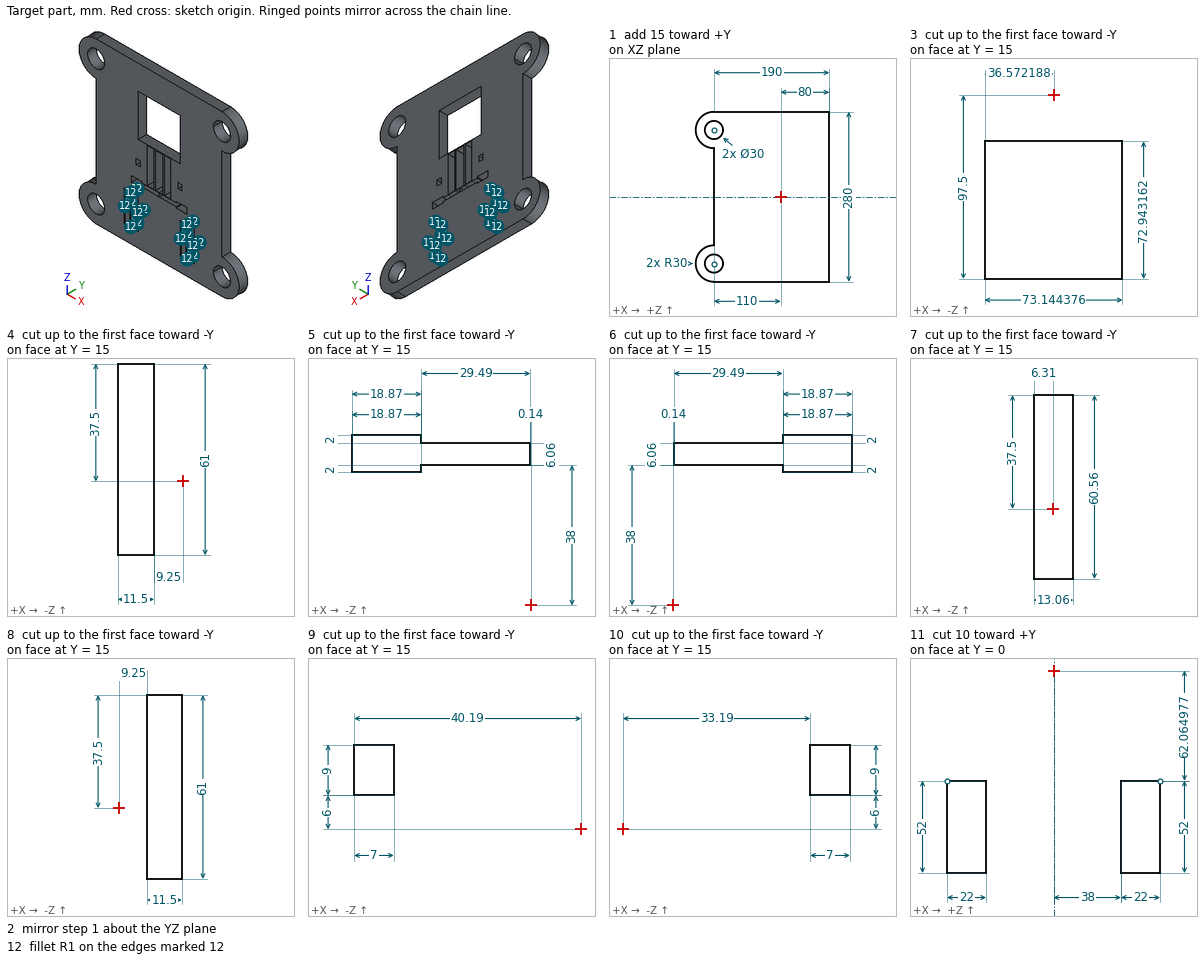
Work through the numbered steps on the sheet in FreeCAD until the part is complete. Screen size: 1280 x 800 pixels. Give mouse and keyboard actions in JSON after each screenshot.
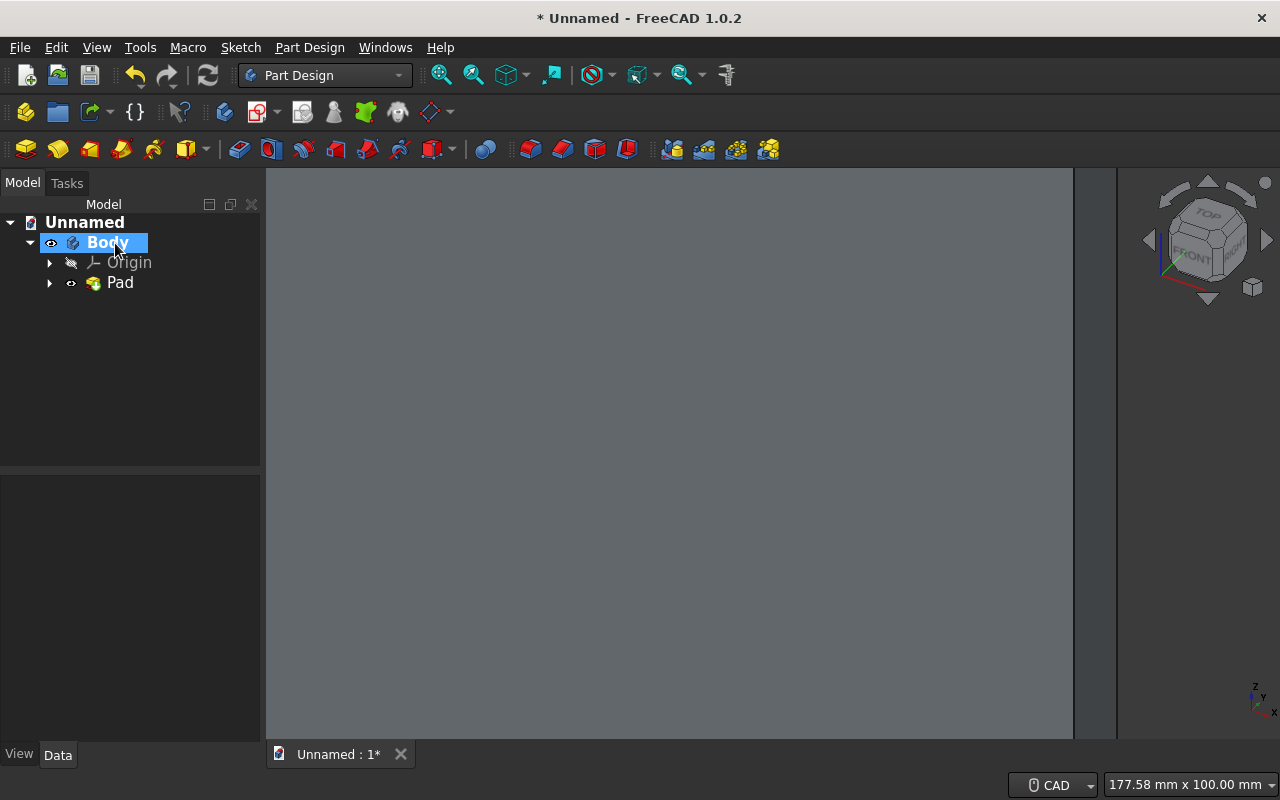
{"action": "left_click", "coordinate": [442, 76]}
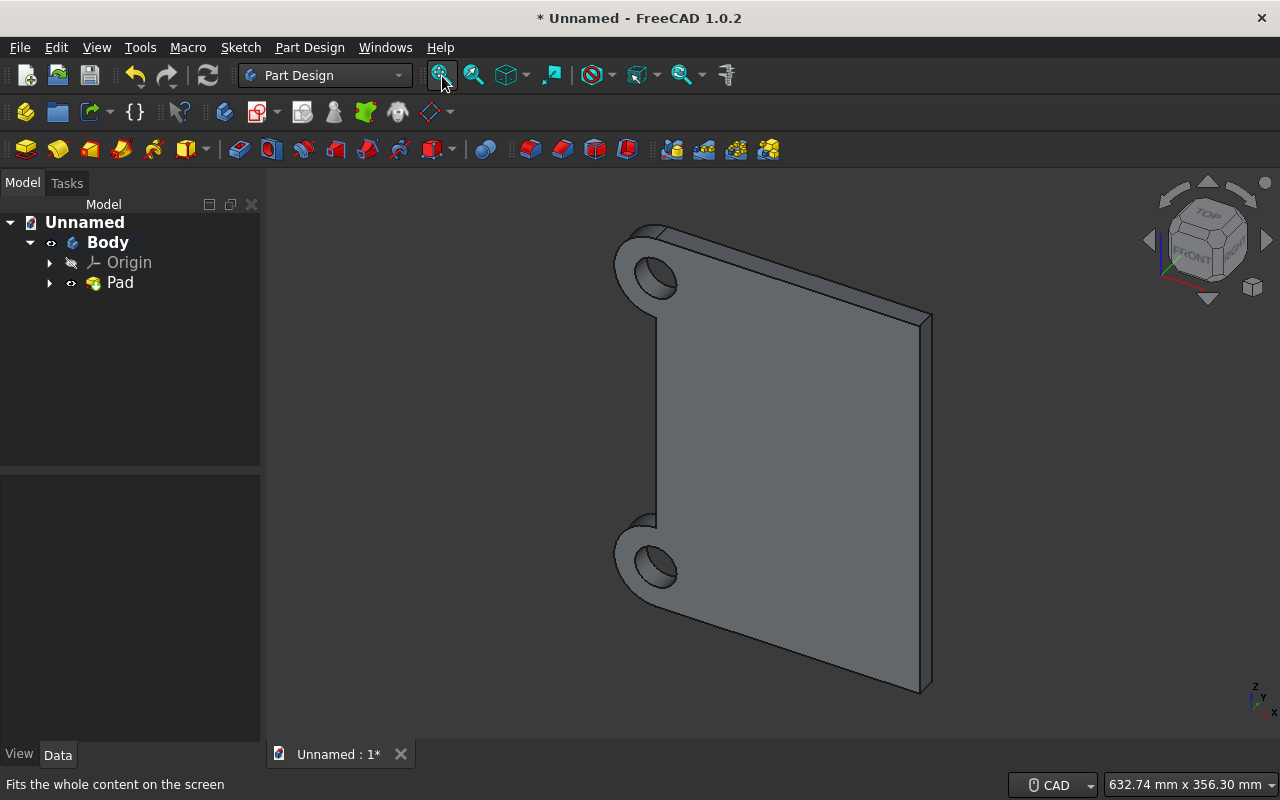
{"action": "left_click", "coordinate": [116, 283]}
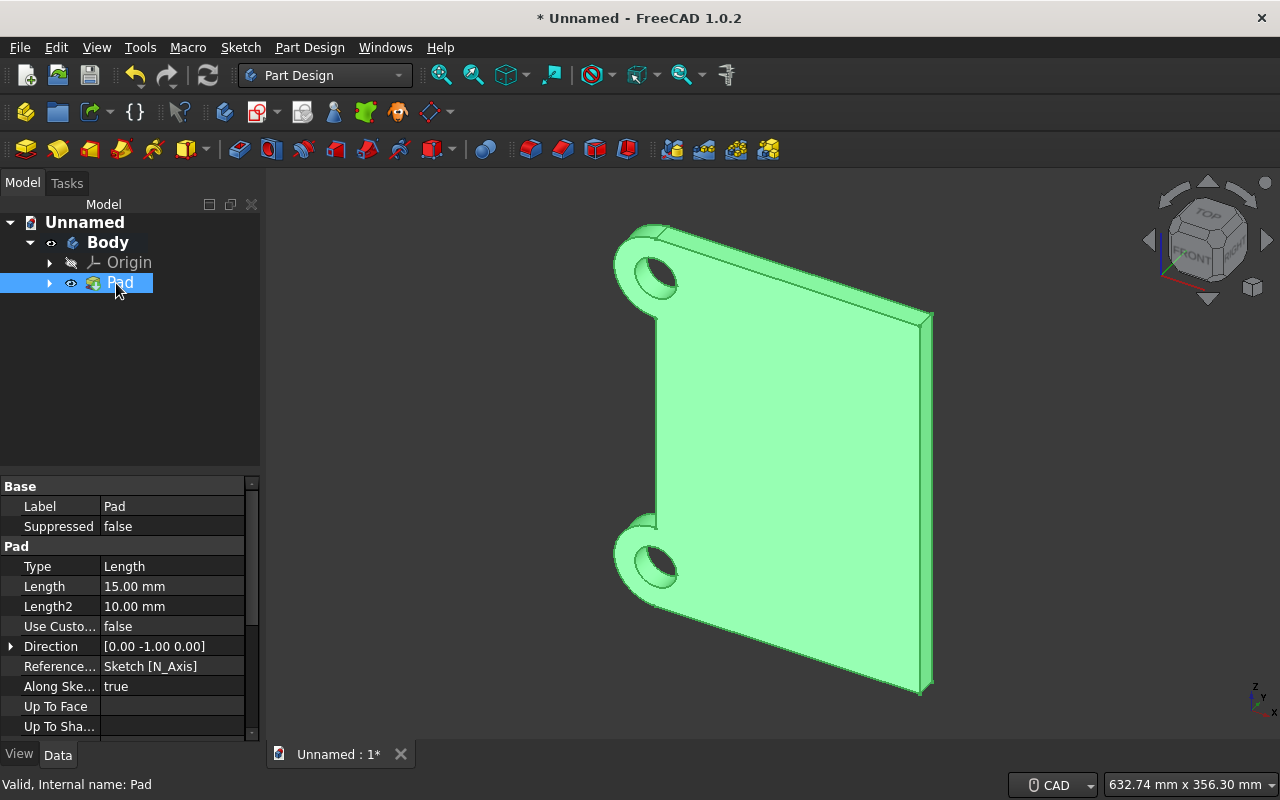
{"action": "left_click", "coordinate": [672, 150]}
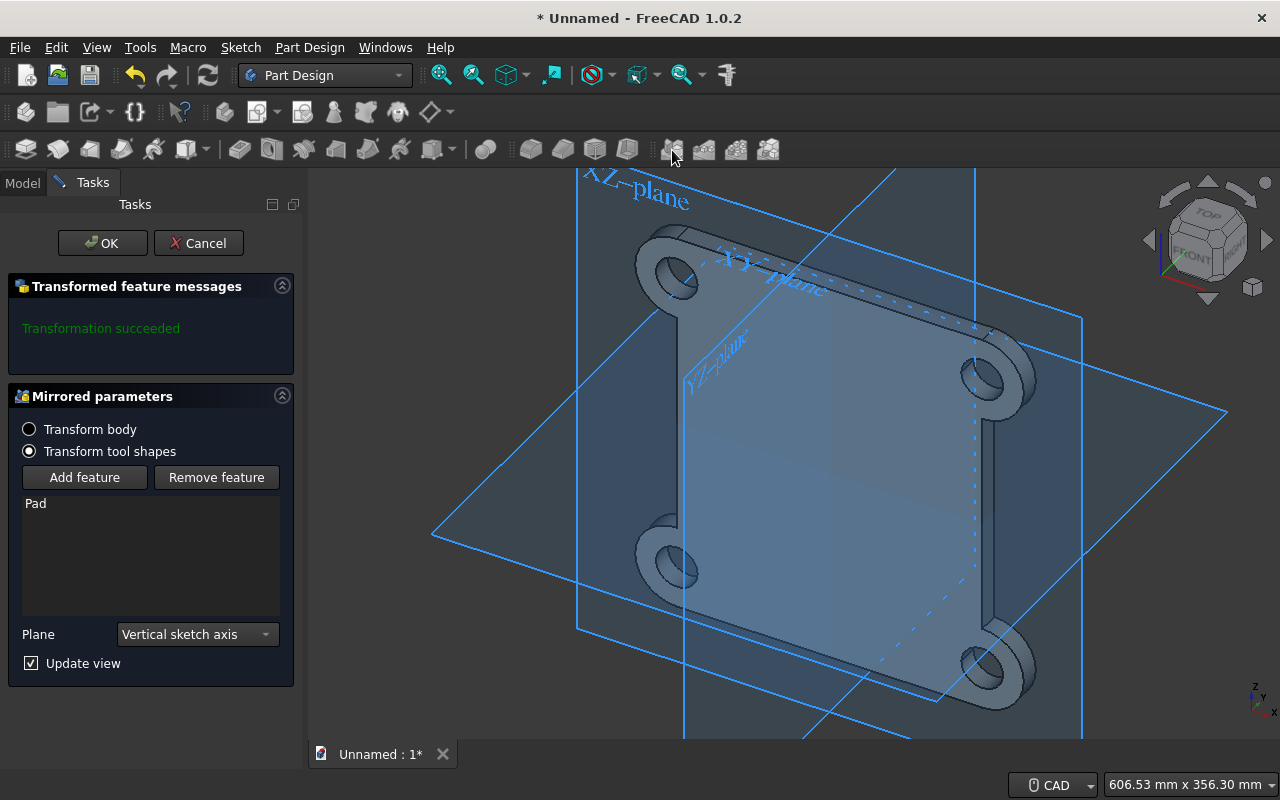
{"action": "left_click", "coordinate": [198, 634]}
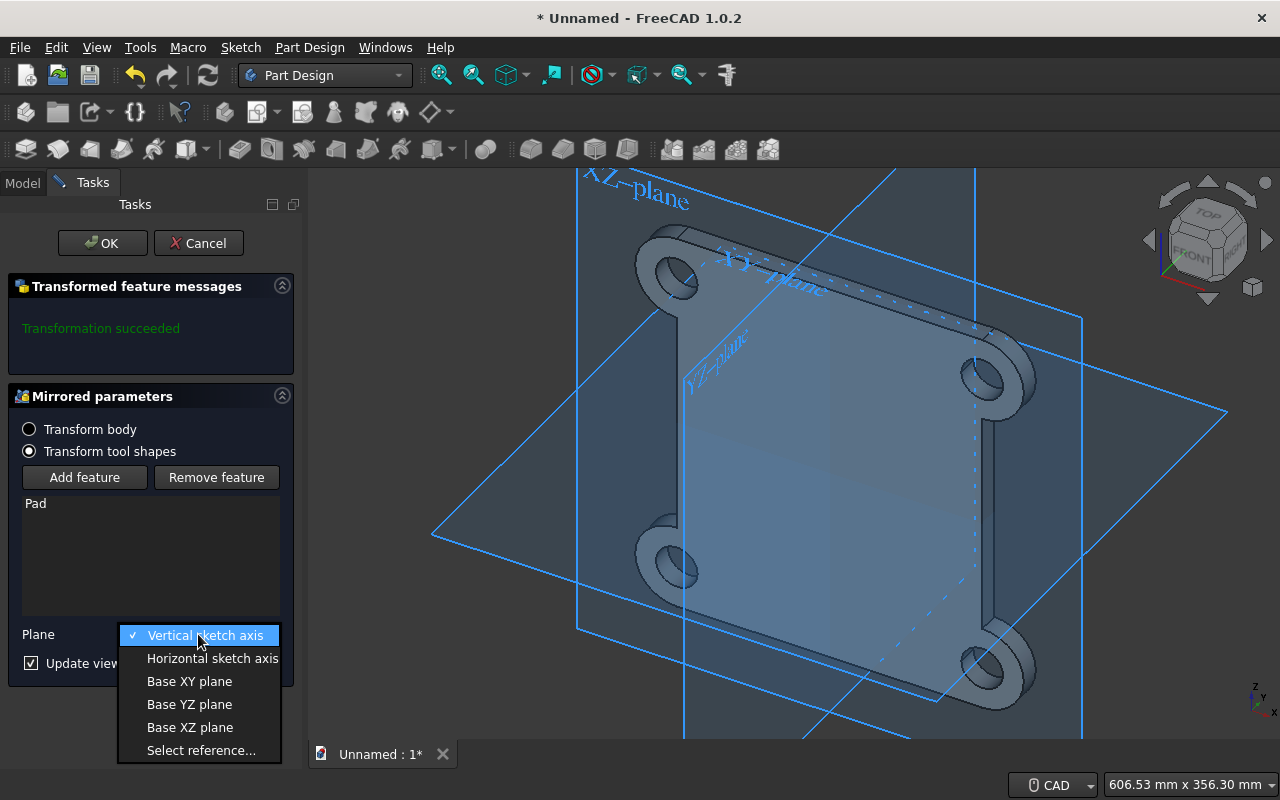
{"action": "left_click", "coordinate": [198, 704]}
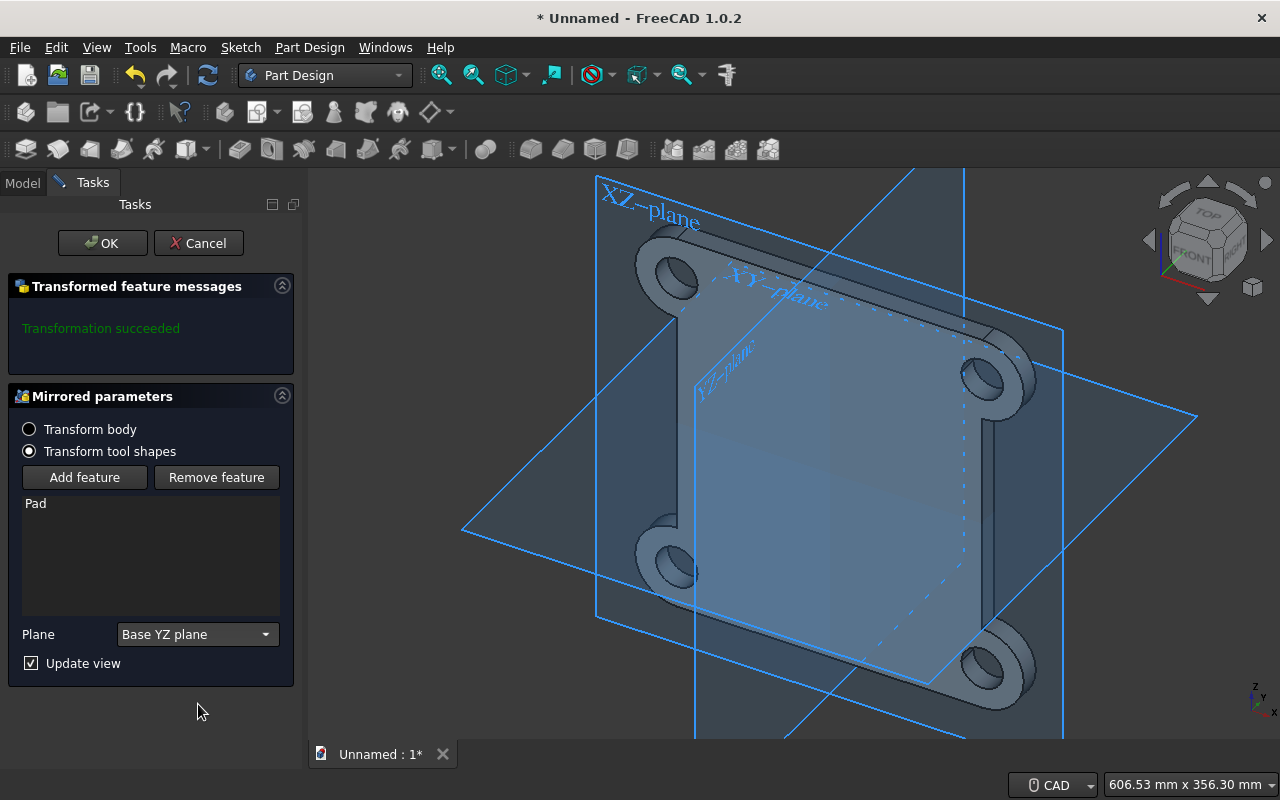
{"action": "left_click", "coordinate": [103, 243]}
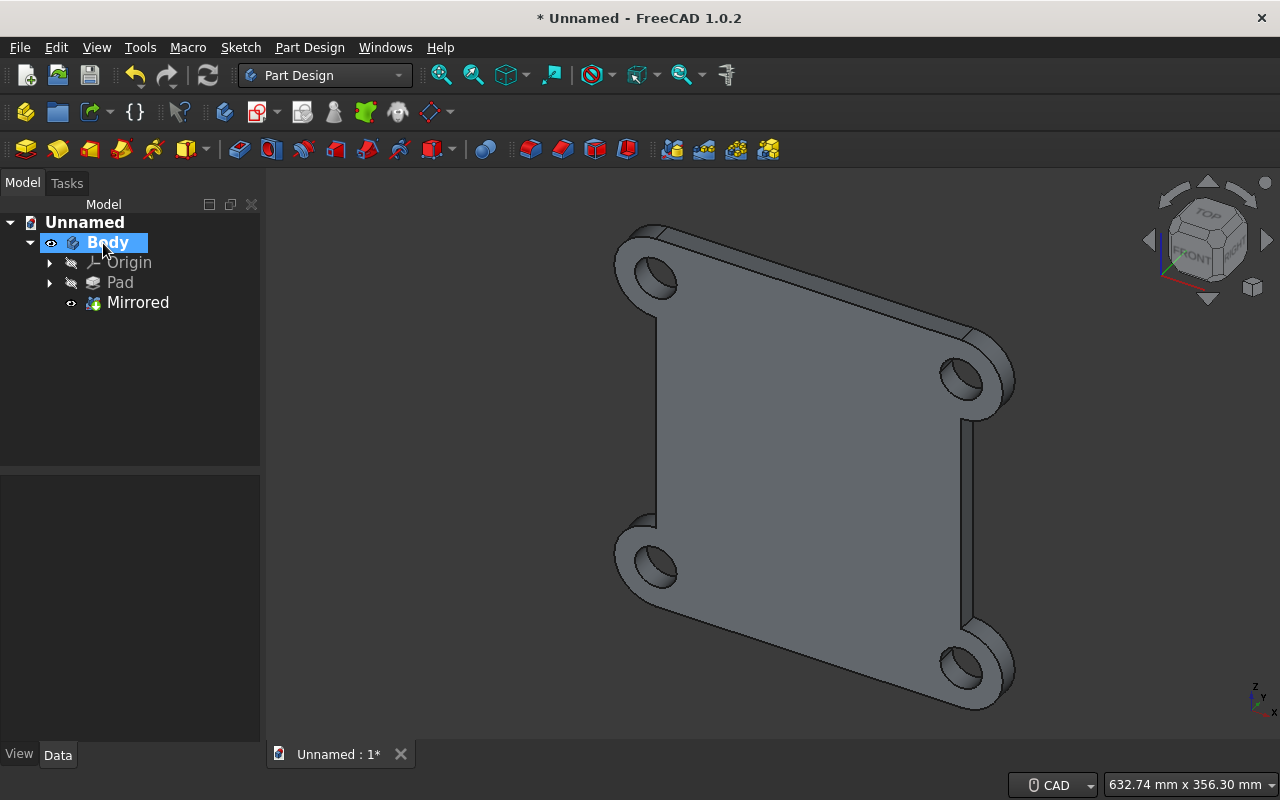
{"action": "key", "text": "4"}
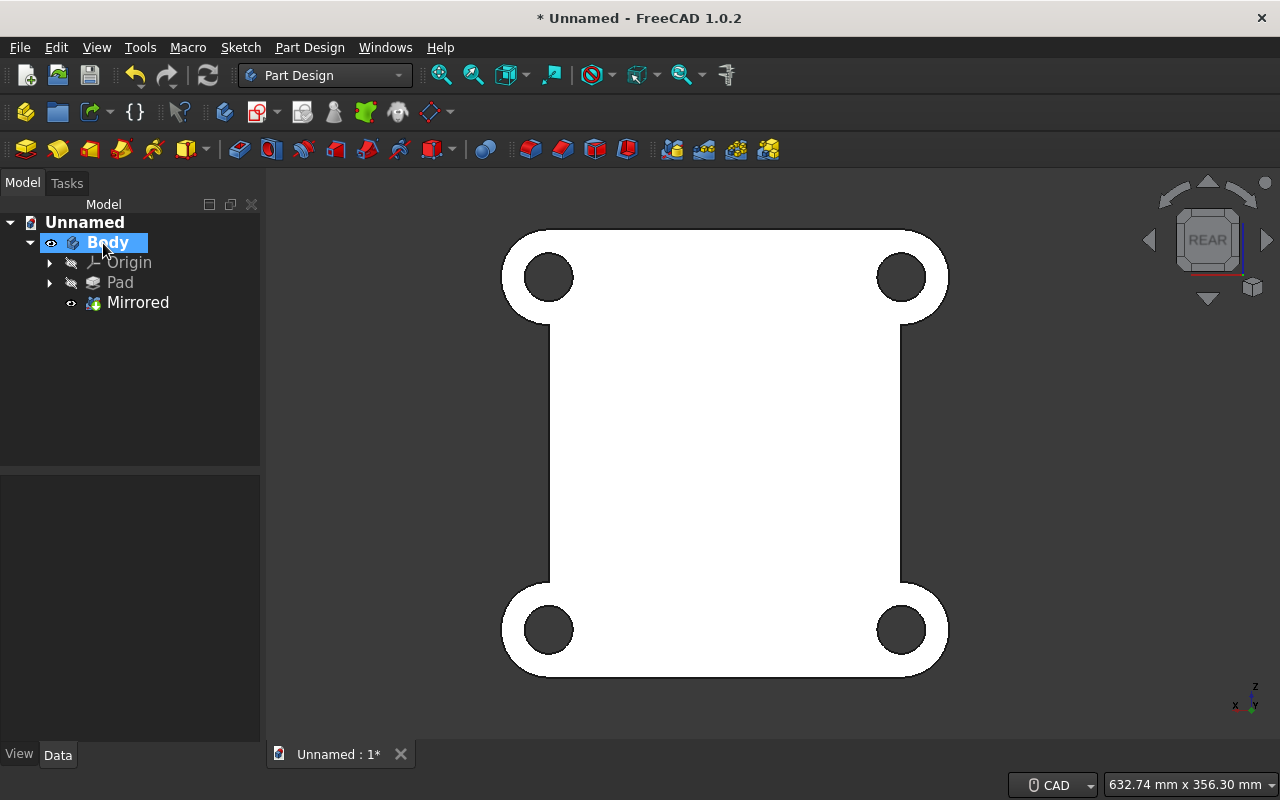
{"action": "left_click", "coordinate": [725, 452]}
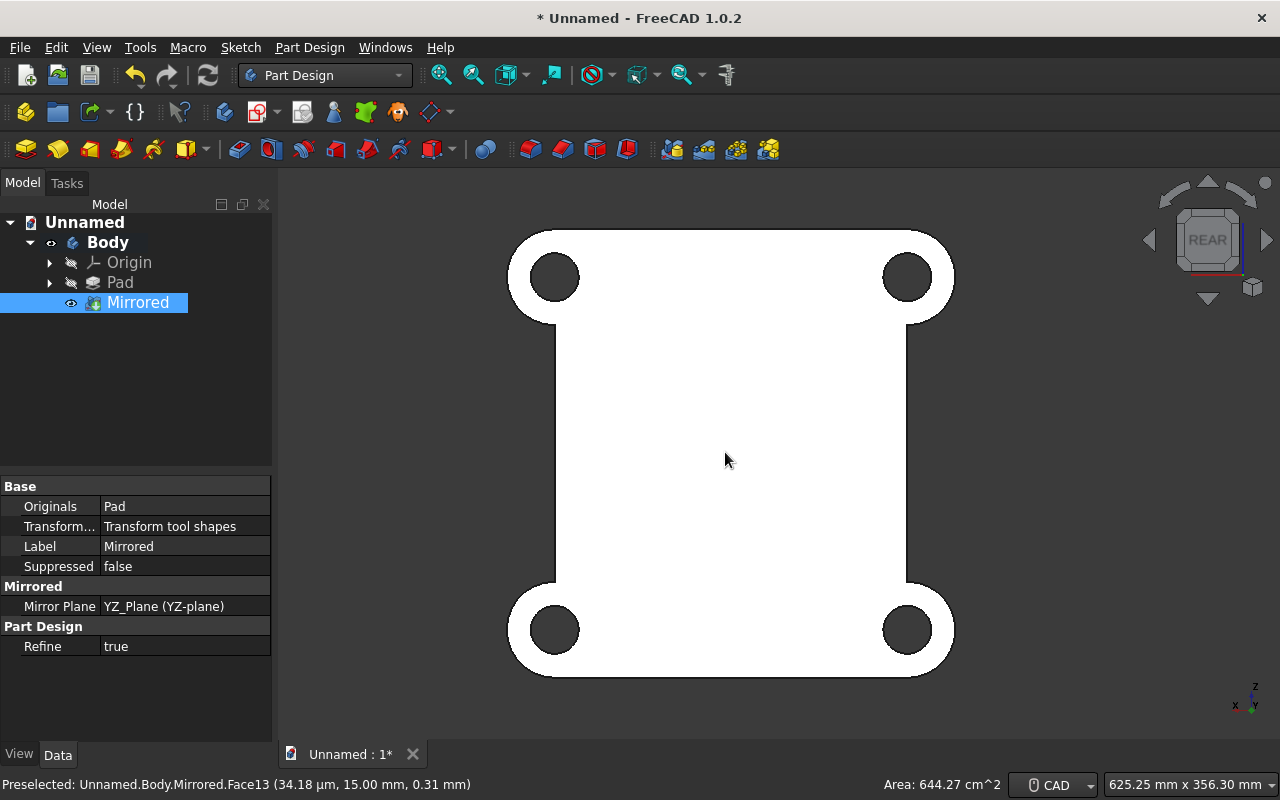
{"action": "left_click", "coordinate": [258, 112]}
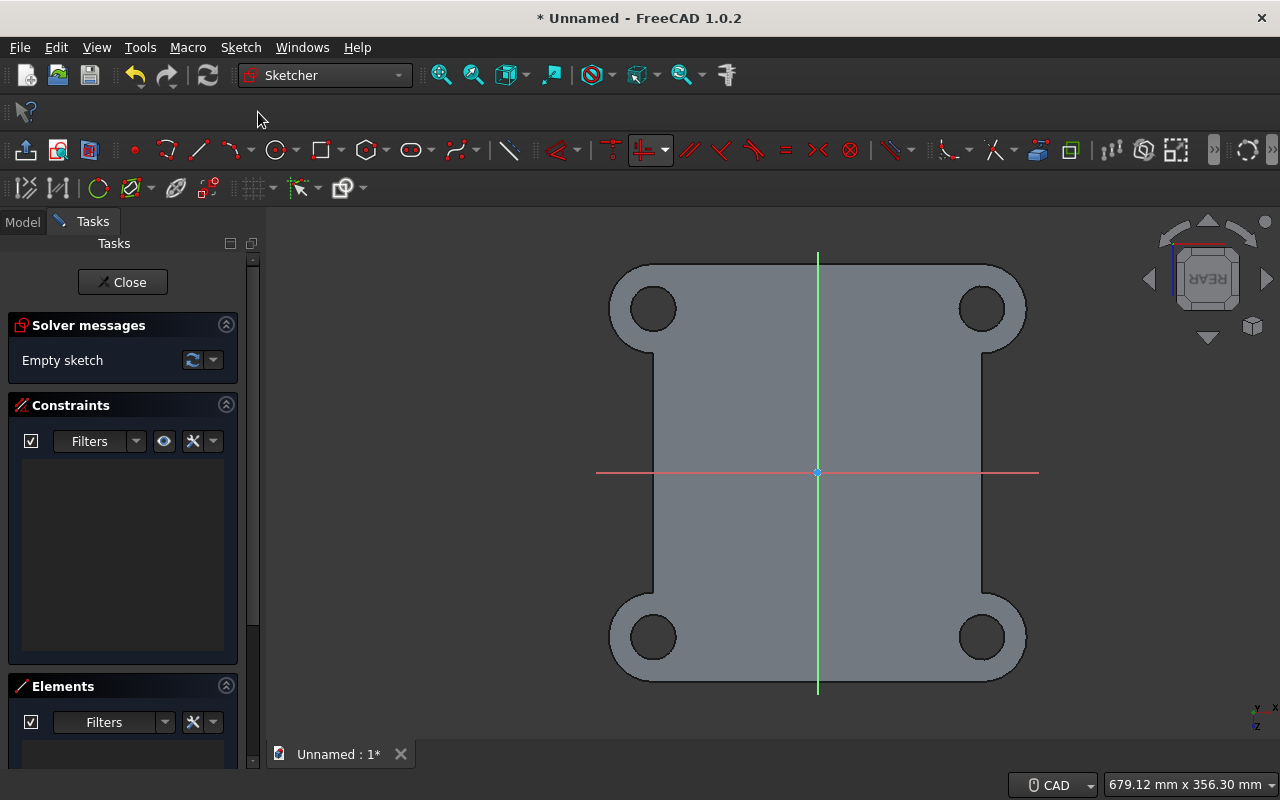
{"action": "scroll", "coordinate": [910, 605], "scroll_direction": "up", "scroll_amount": 4}